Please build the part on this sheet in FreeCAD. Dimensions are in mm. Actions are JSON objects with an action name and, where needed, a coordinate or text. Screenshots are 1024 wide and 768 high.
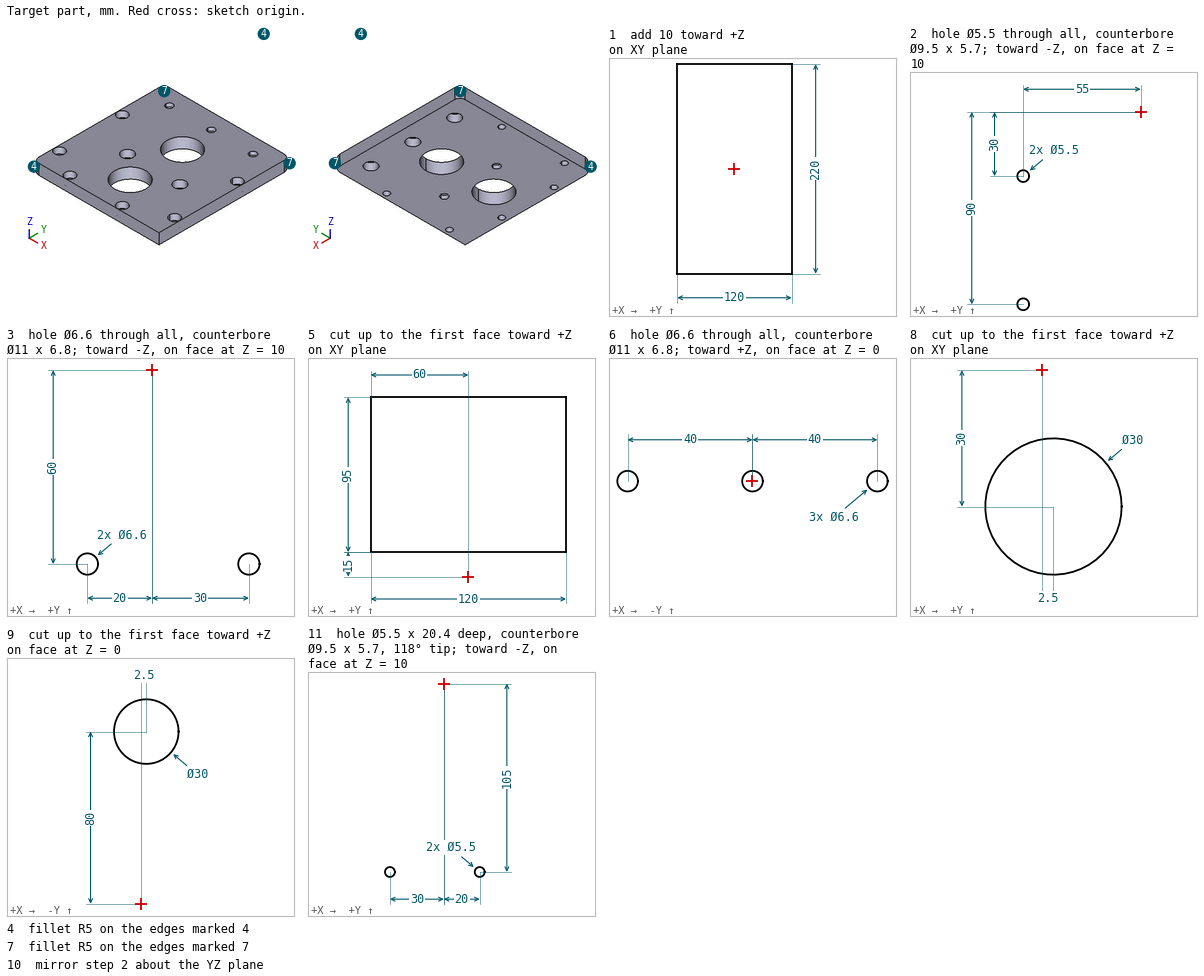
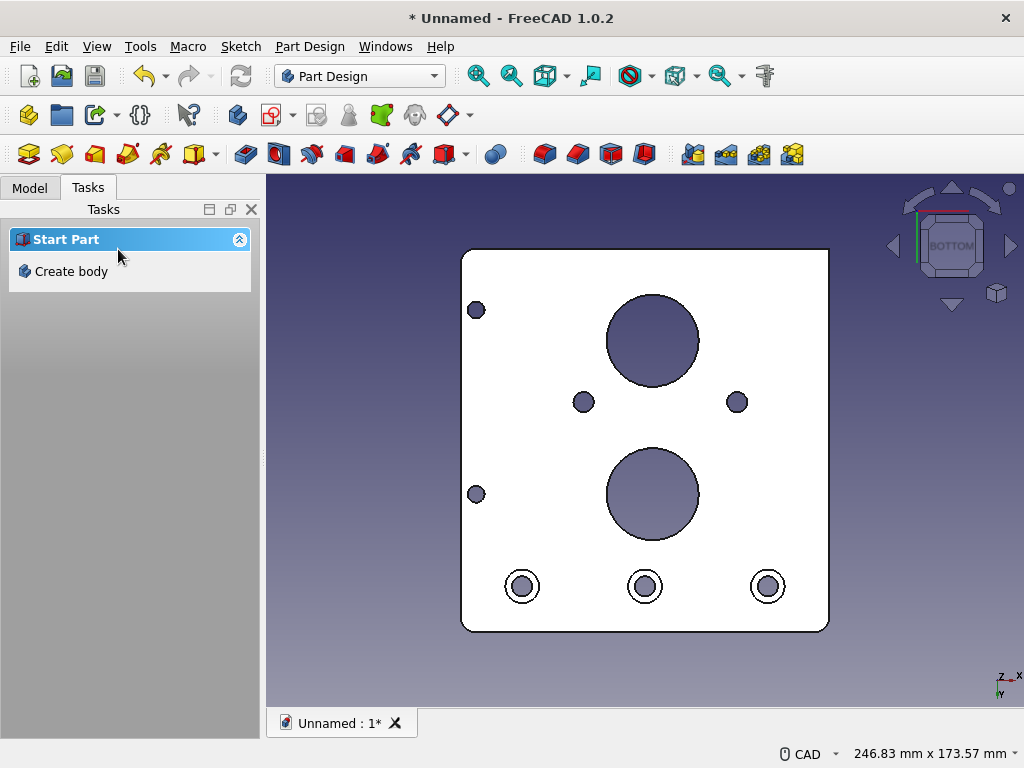
{"action": "left_click", "coordinate": [30, 188]}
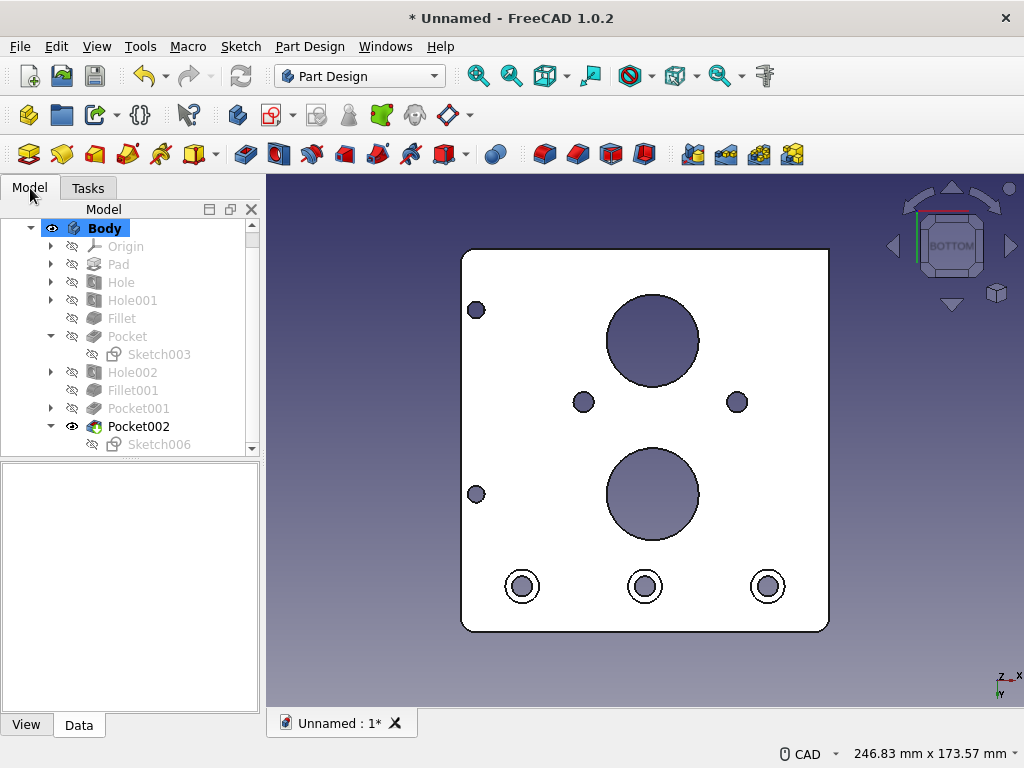
{"action": "left_click", "coordinate": [117, 282]}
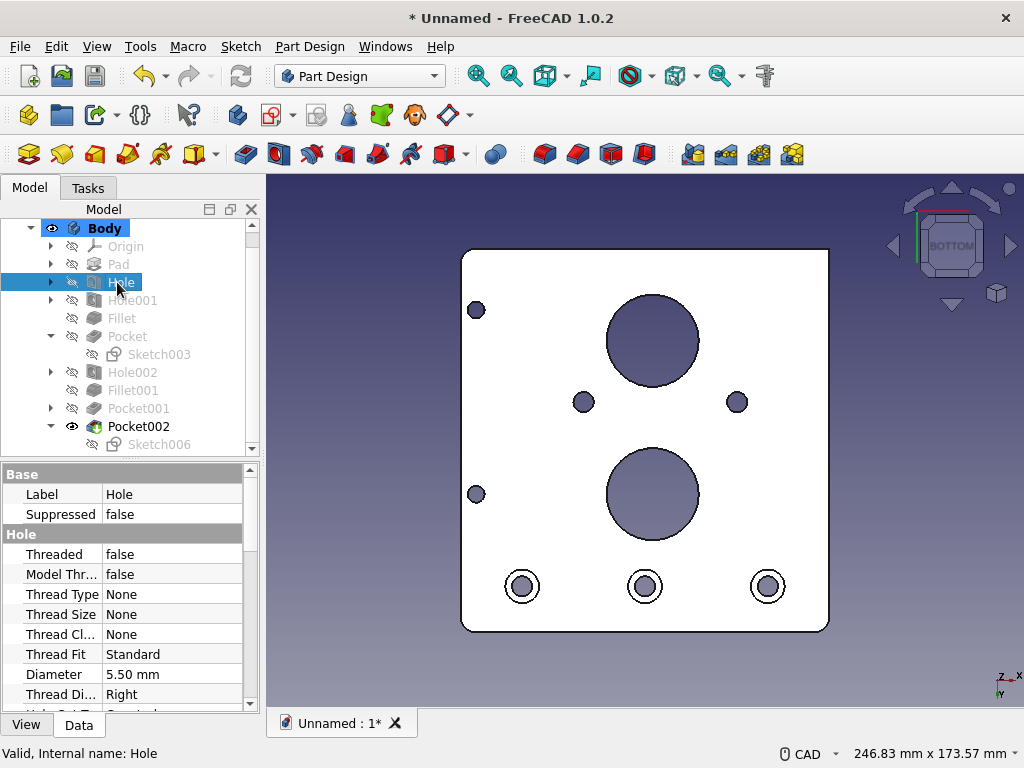
{"action": "left_click", "coordinate": [693, 154]}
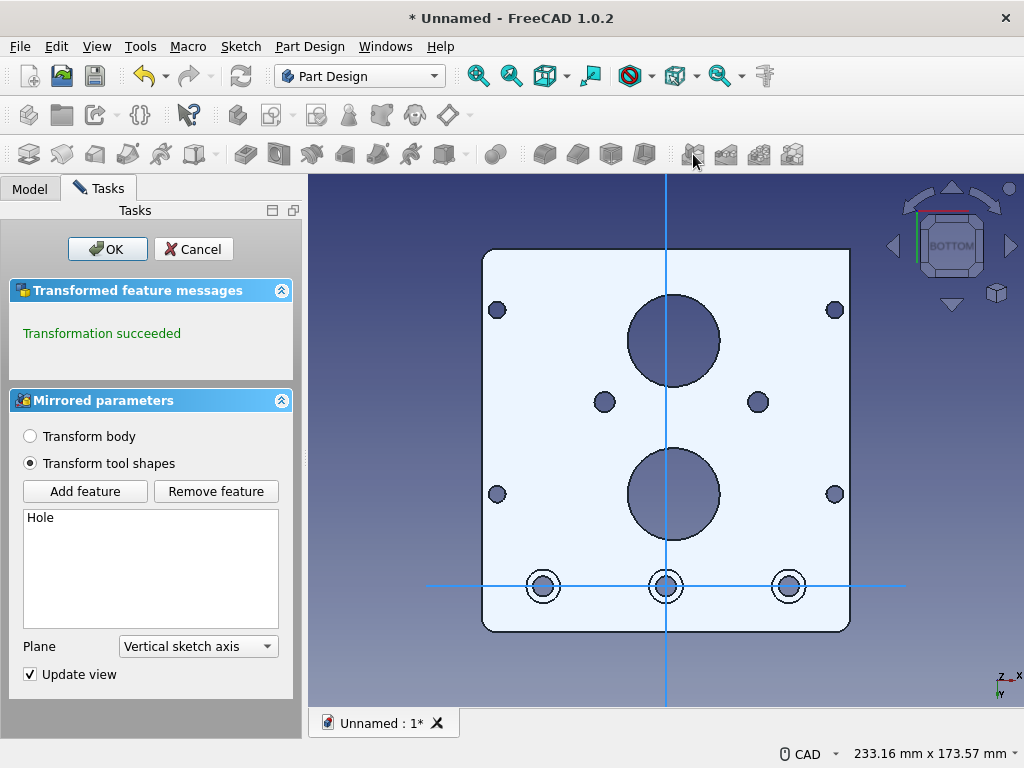
{"action": "left_click", "coordinate": [199, 646]}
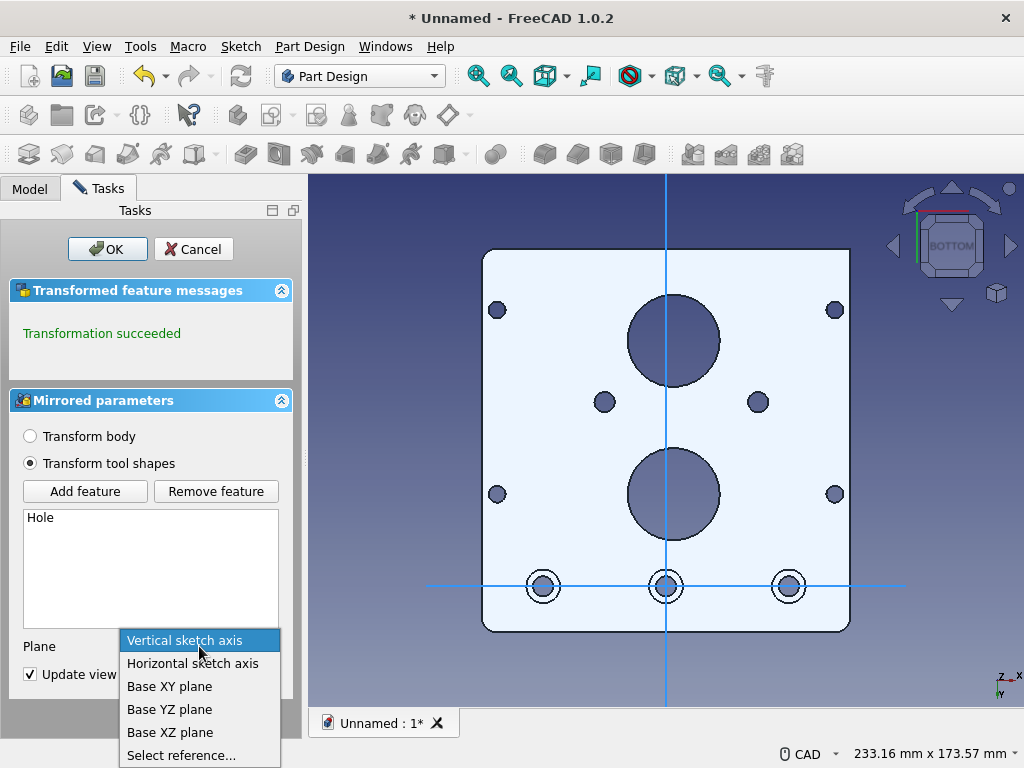
{"action": "left_click", "coordinate": [198, 710]}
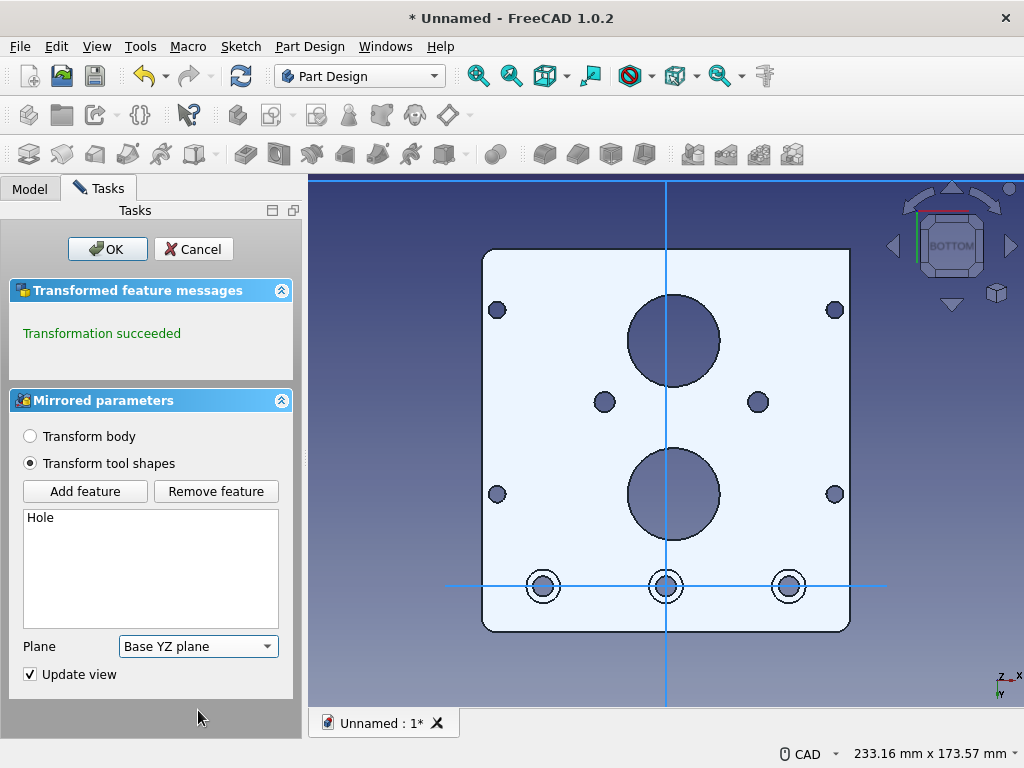
{"action": "left_click", "coordinate": [108, 249]}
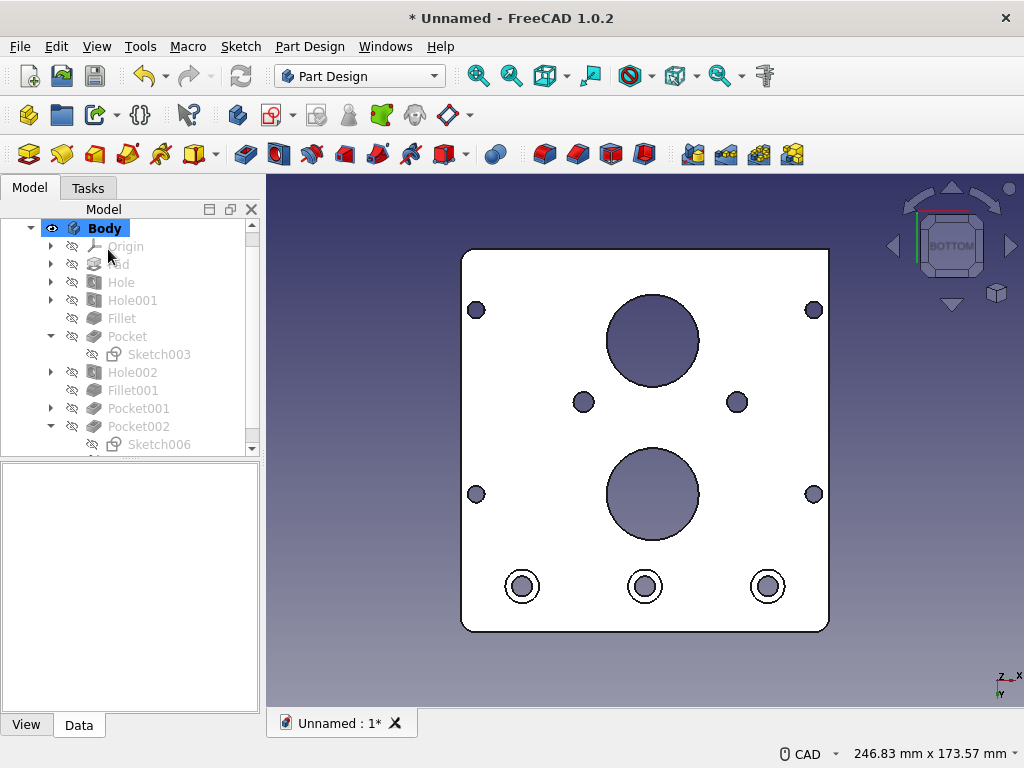
{"action": "key", "text": "0"}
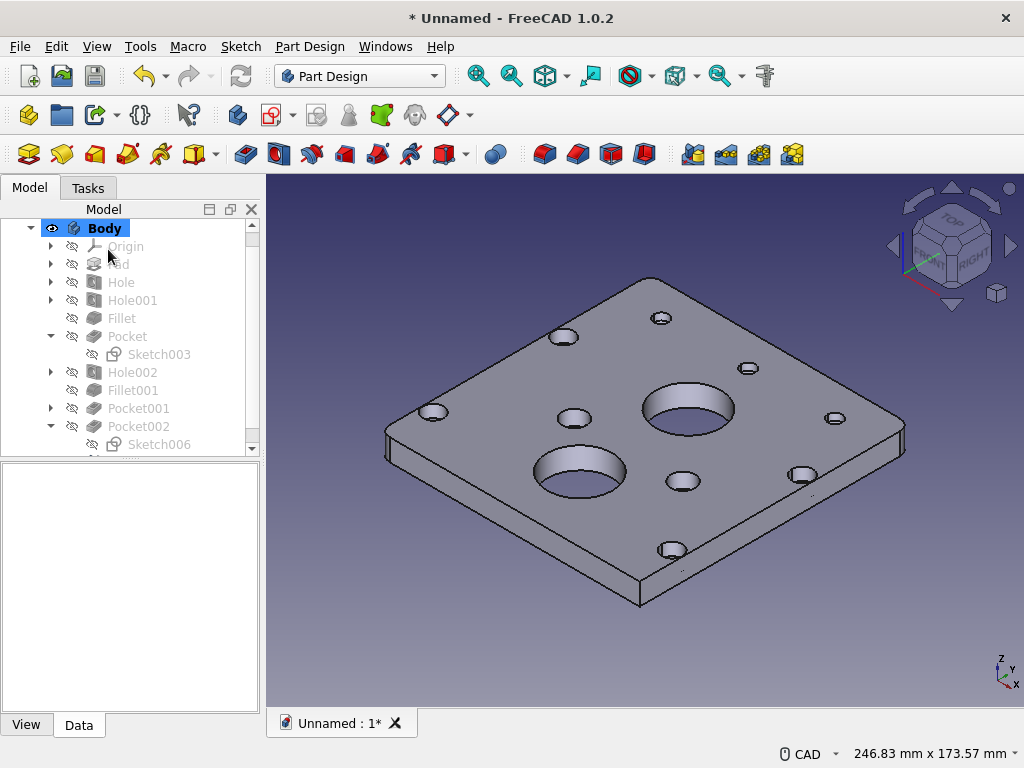
{"action": "left_click", "coordinate": [493, 429]}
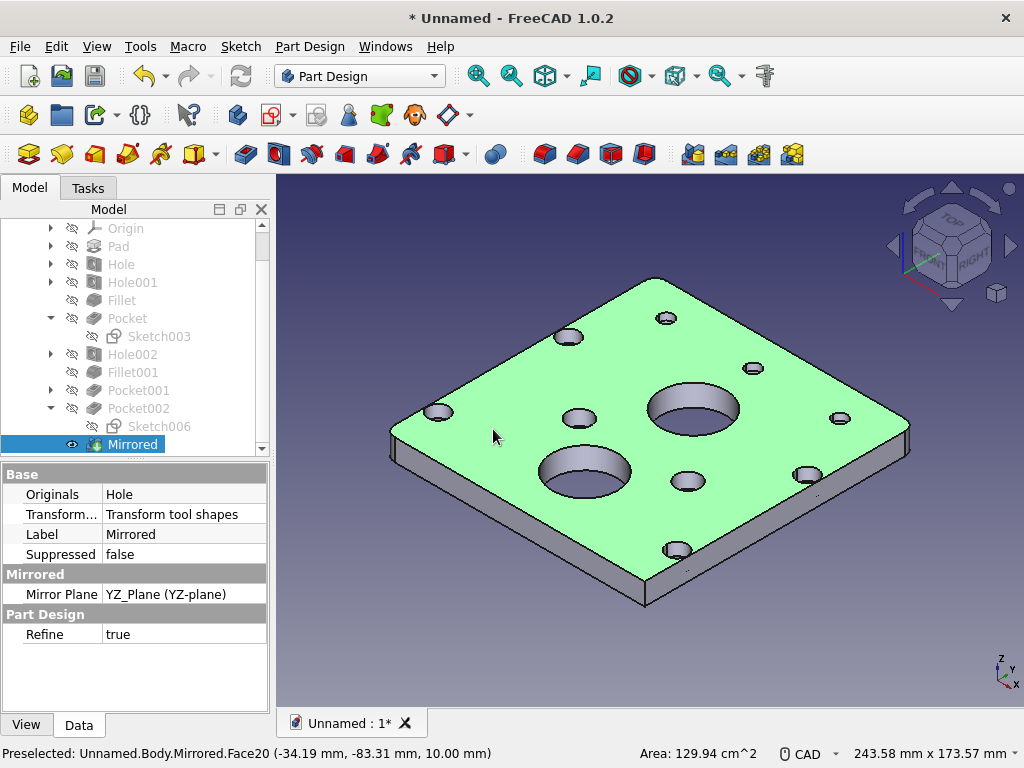
{"action": "left_click", "coordinate": [270, 116]}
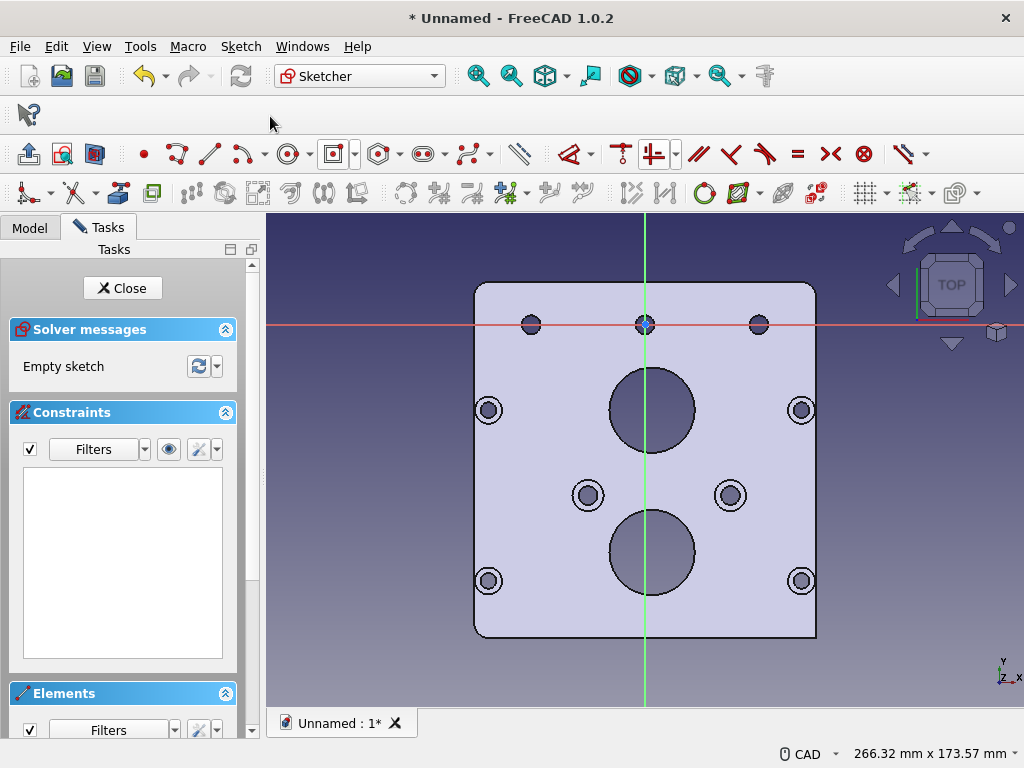
{"action": "left_click", "coordinate": [288, 154]}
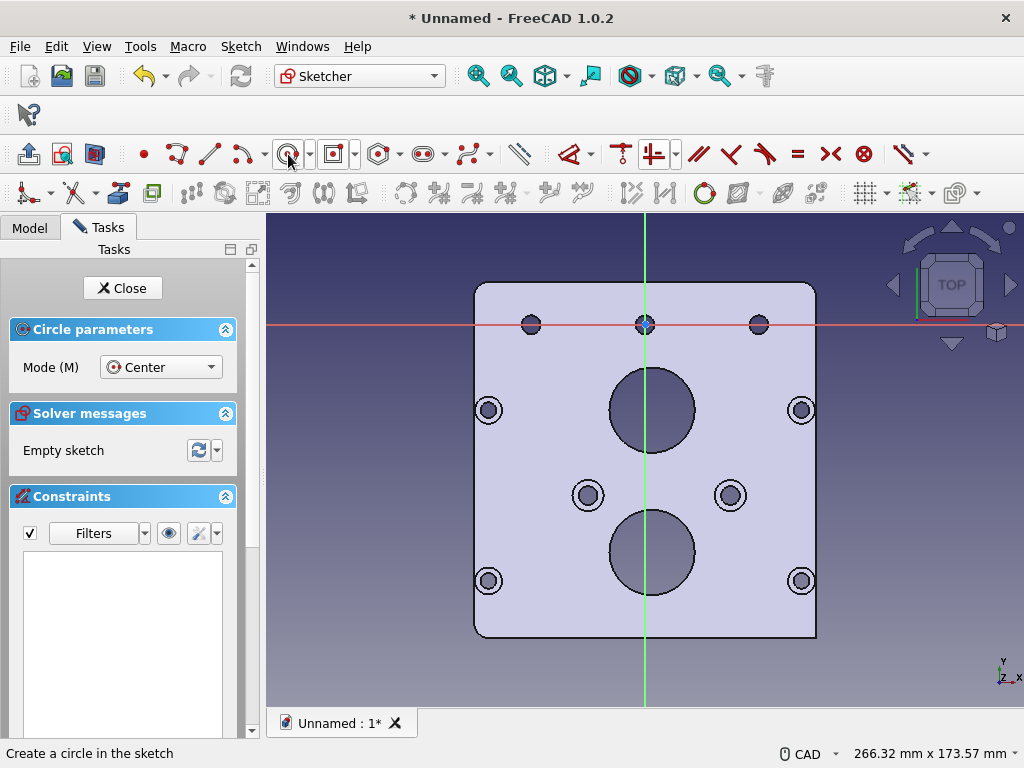
{"action": "scroll", "coordinate": [702, 624], "scroll_direction": "up", "scroll_amount": 6}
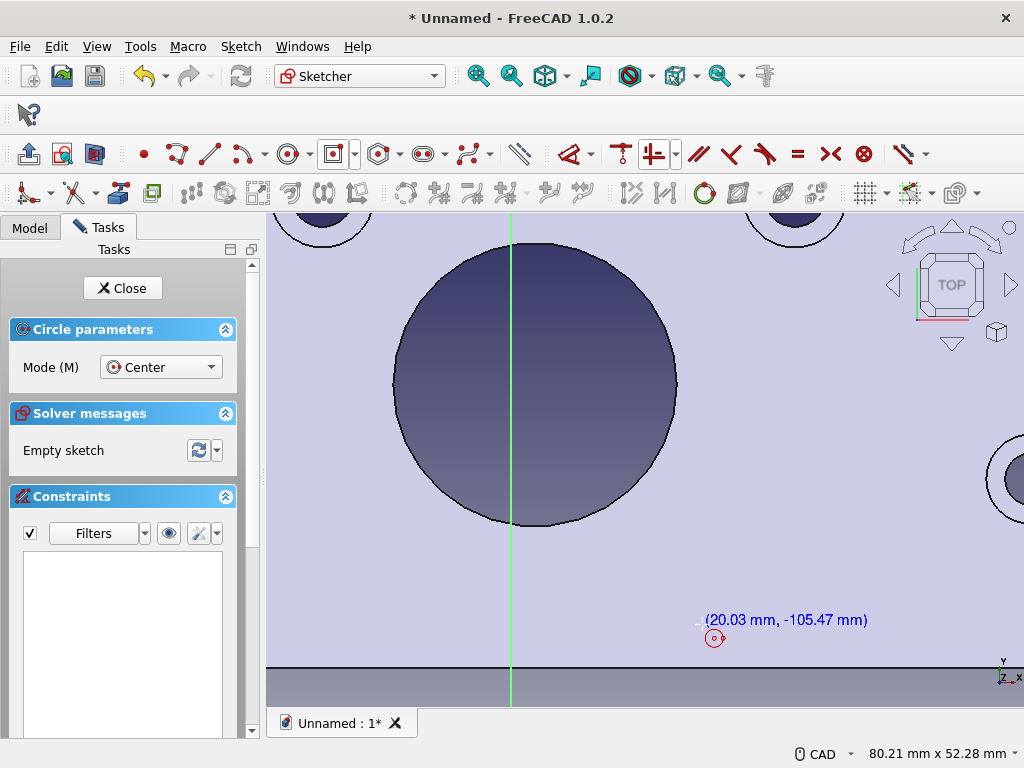
{"action": "left_click", "coordinate": [700, 621]}
{"action": "left_click", "coordinate": [719, 603]}